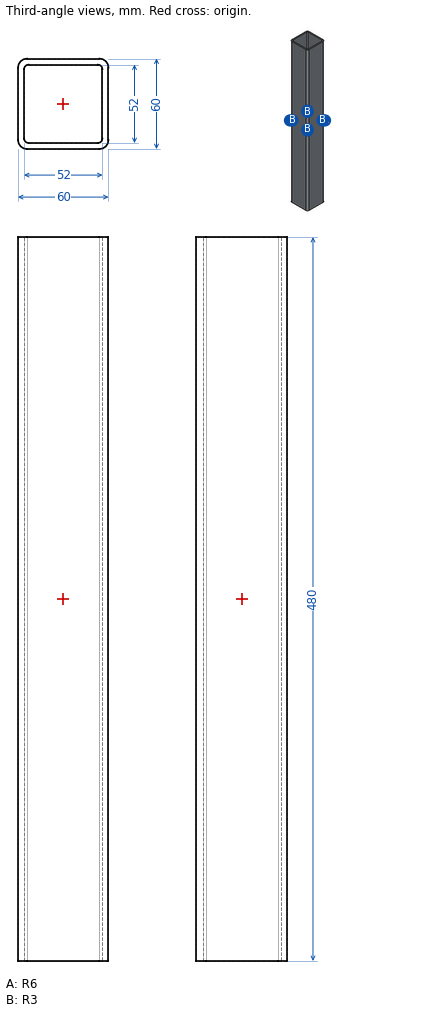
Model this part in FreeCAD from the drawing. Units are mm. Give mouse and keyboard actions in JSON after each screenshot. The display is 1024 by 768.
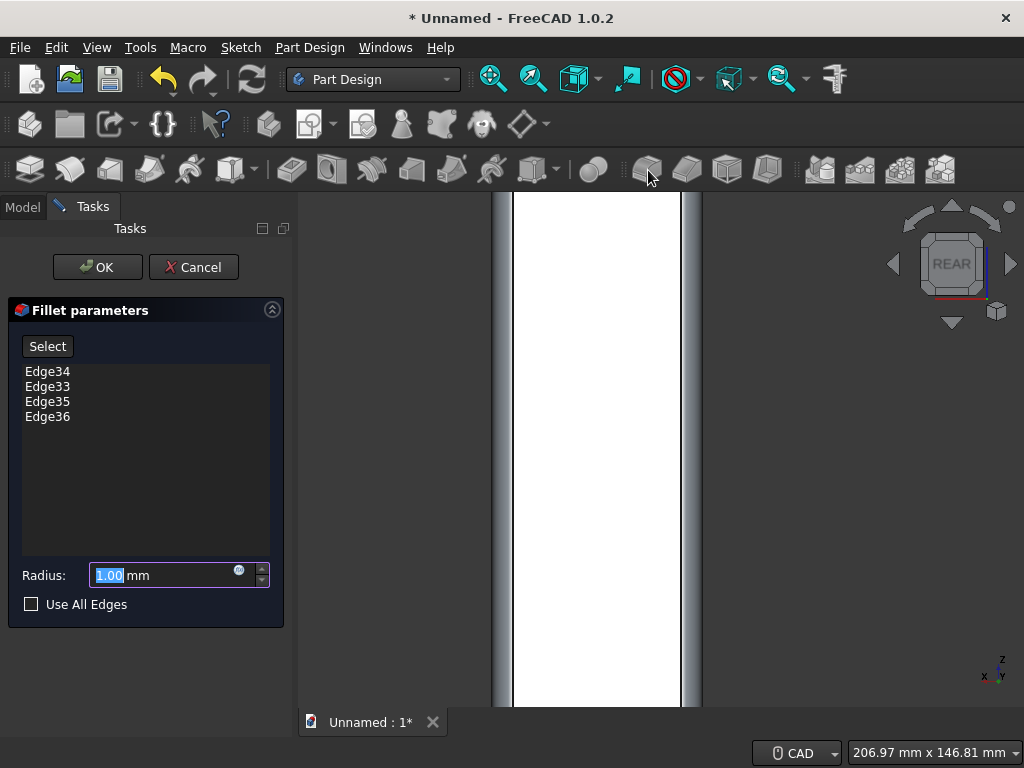
{"action": "type", "text": "3"}
{"action": "key", "text": "Tab"}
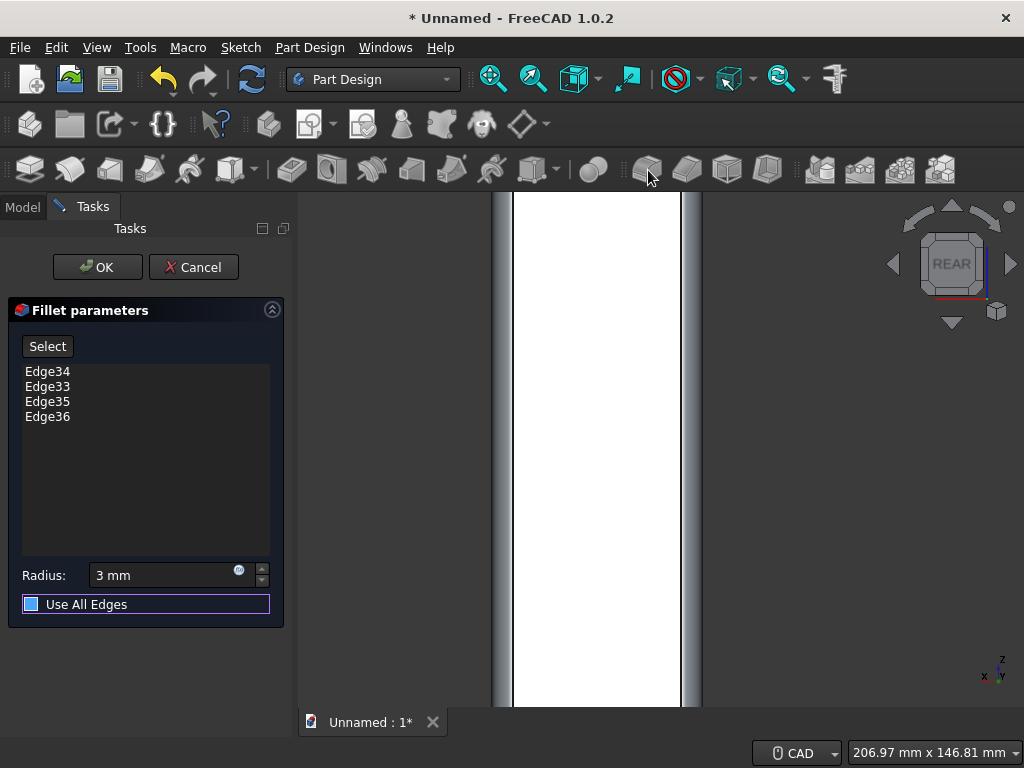
{"action": "left_click", "coordinate": [98, 267]}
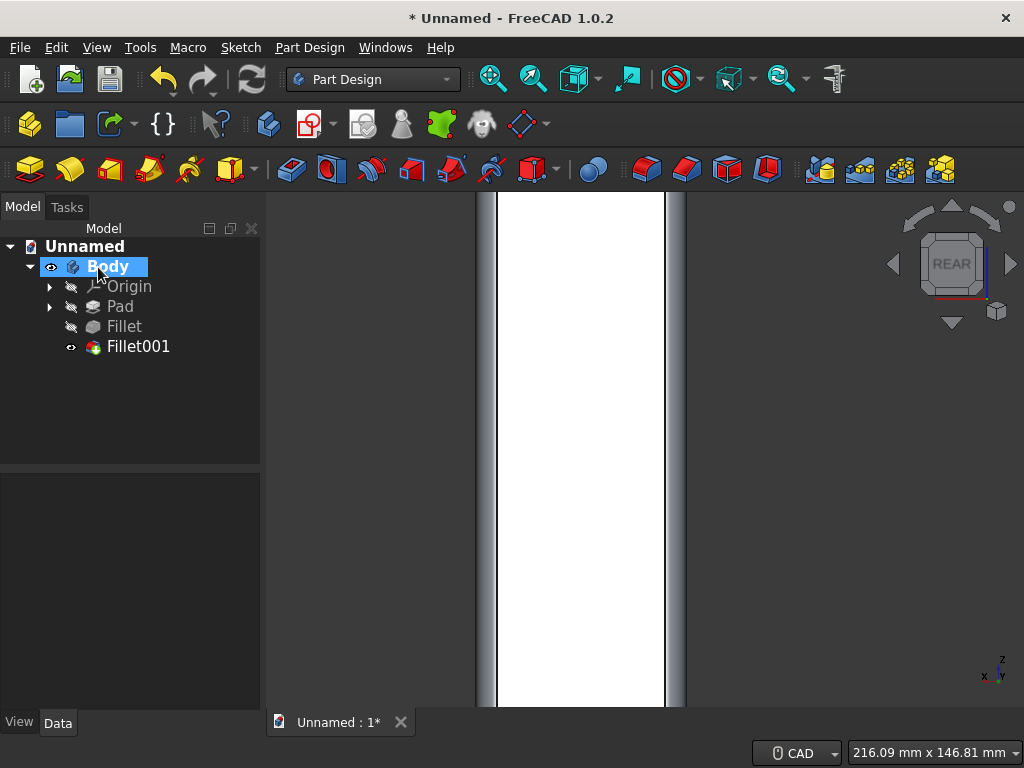
{"action": "key", "text": "0"}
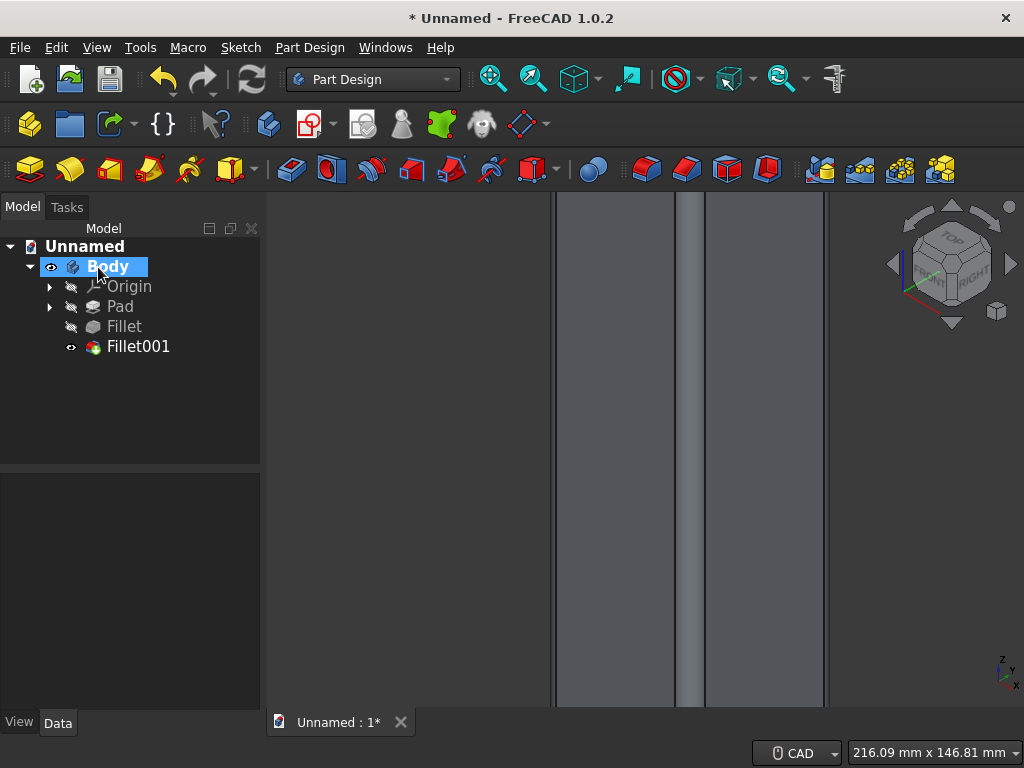
{"action": "left_click", "coordinate": [494, 80]}